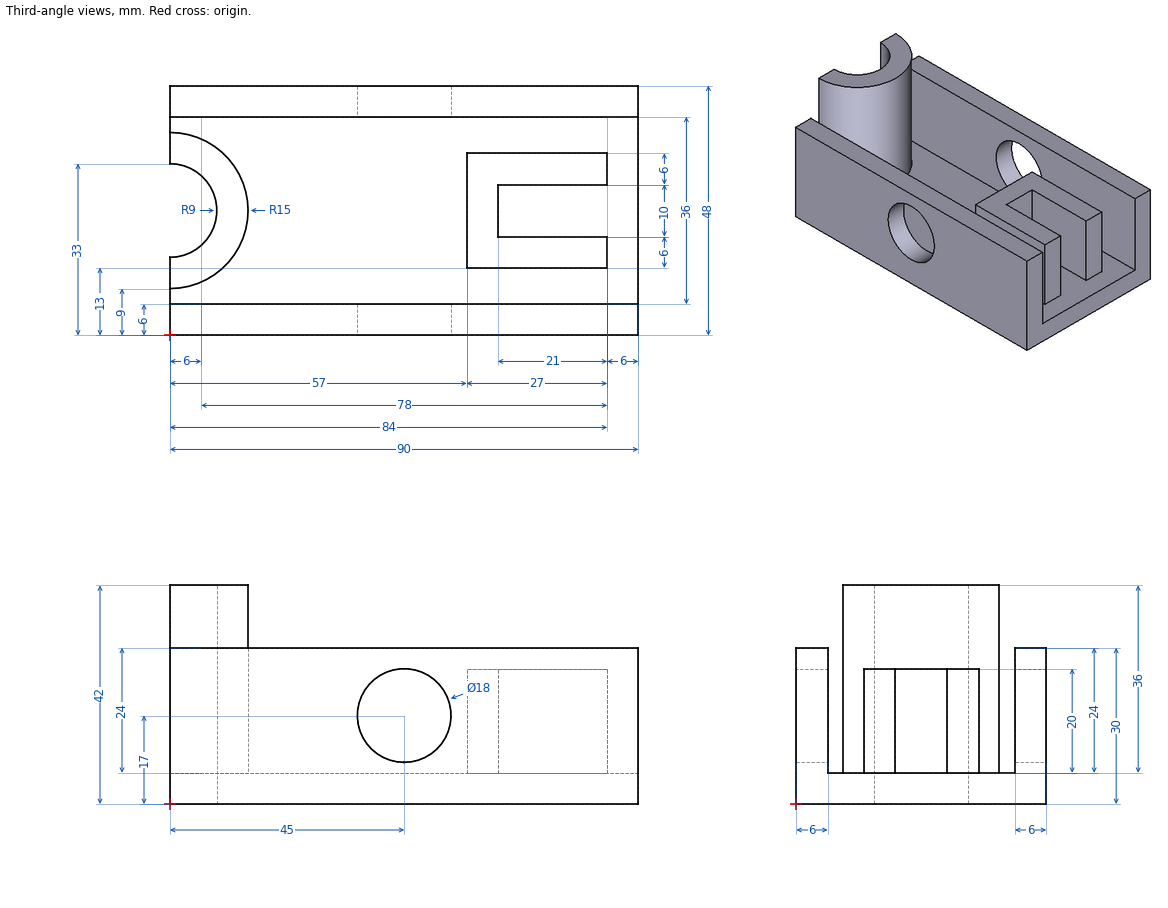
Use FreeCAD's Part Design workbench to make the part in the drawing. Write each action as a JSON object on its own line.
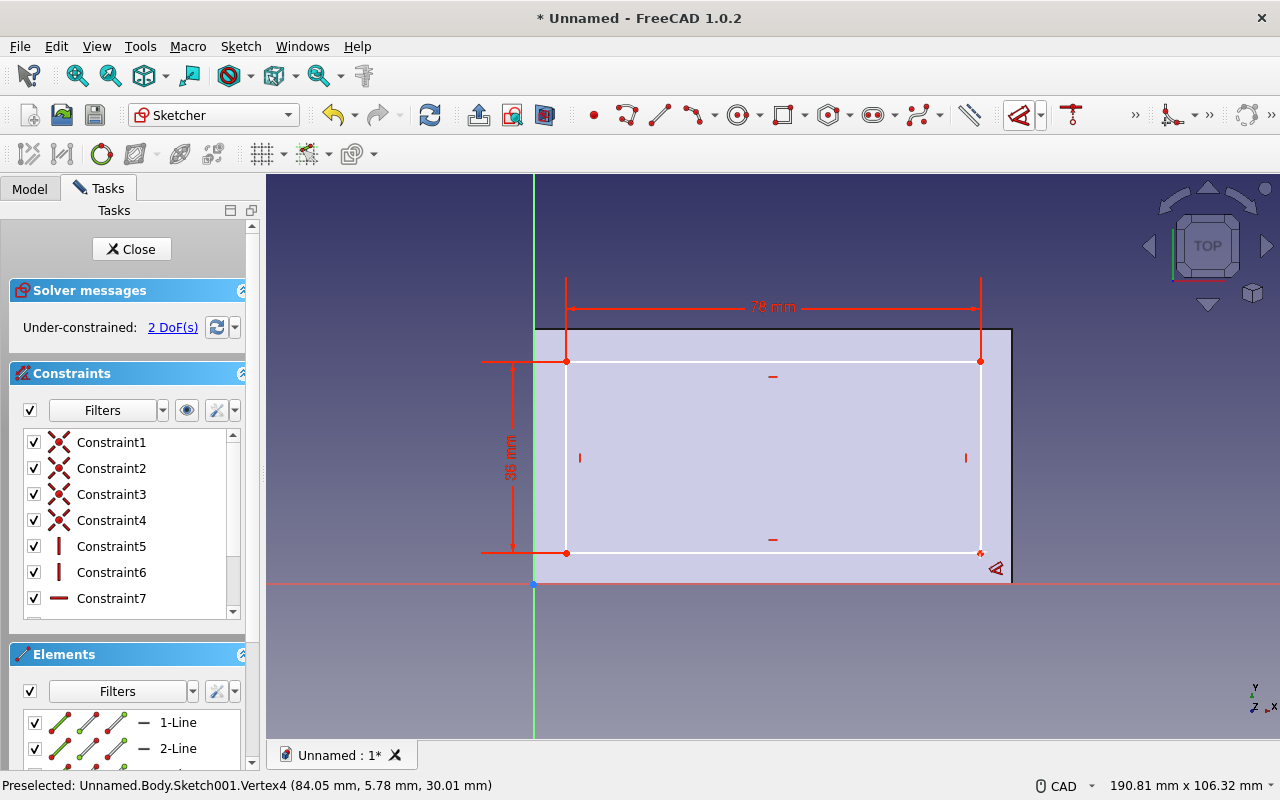
{"action": "scroll", "coordinate": [566, 362], "scroll_direction": "up", "scroll_amount": 2}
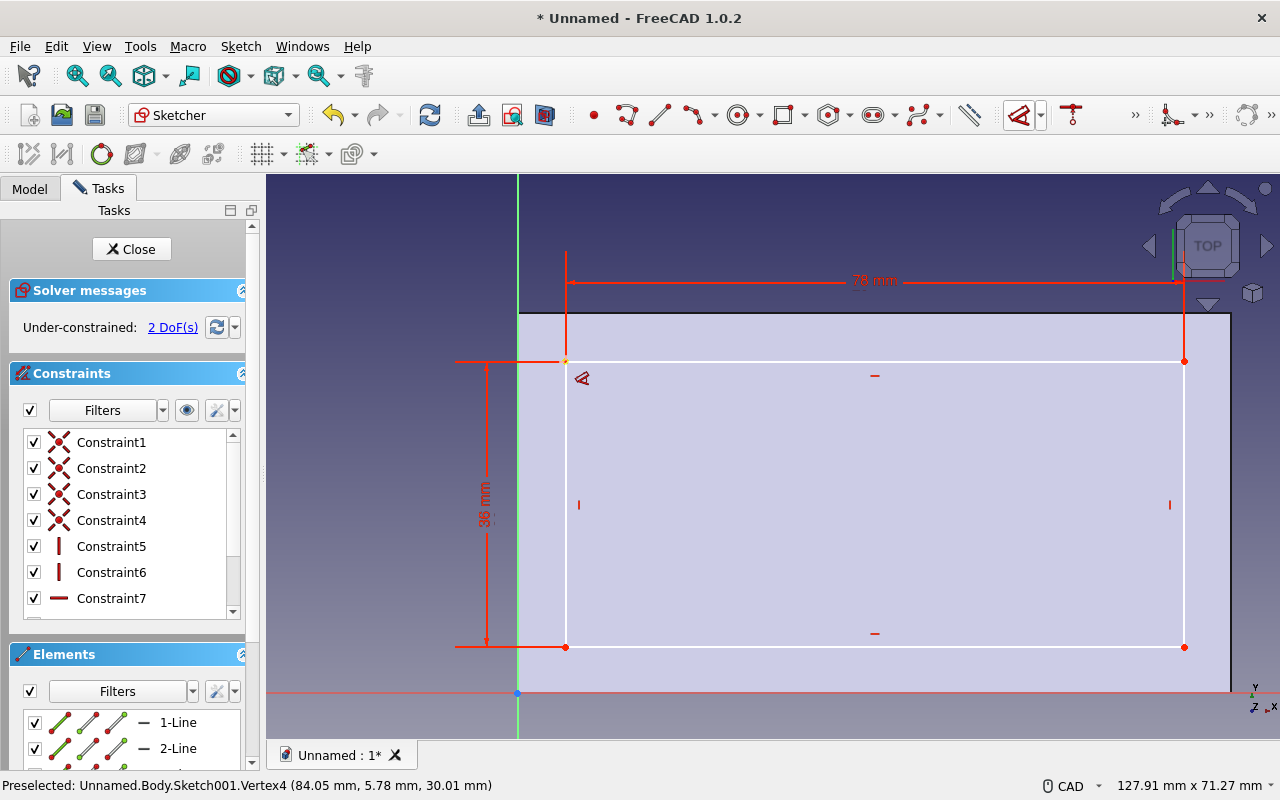
{"action": "left_click", "coordinate": [566, 362]}
{"action": "left_click", "coordinate": [542, 328]}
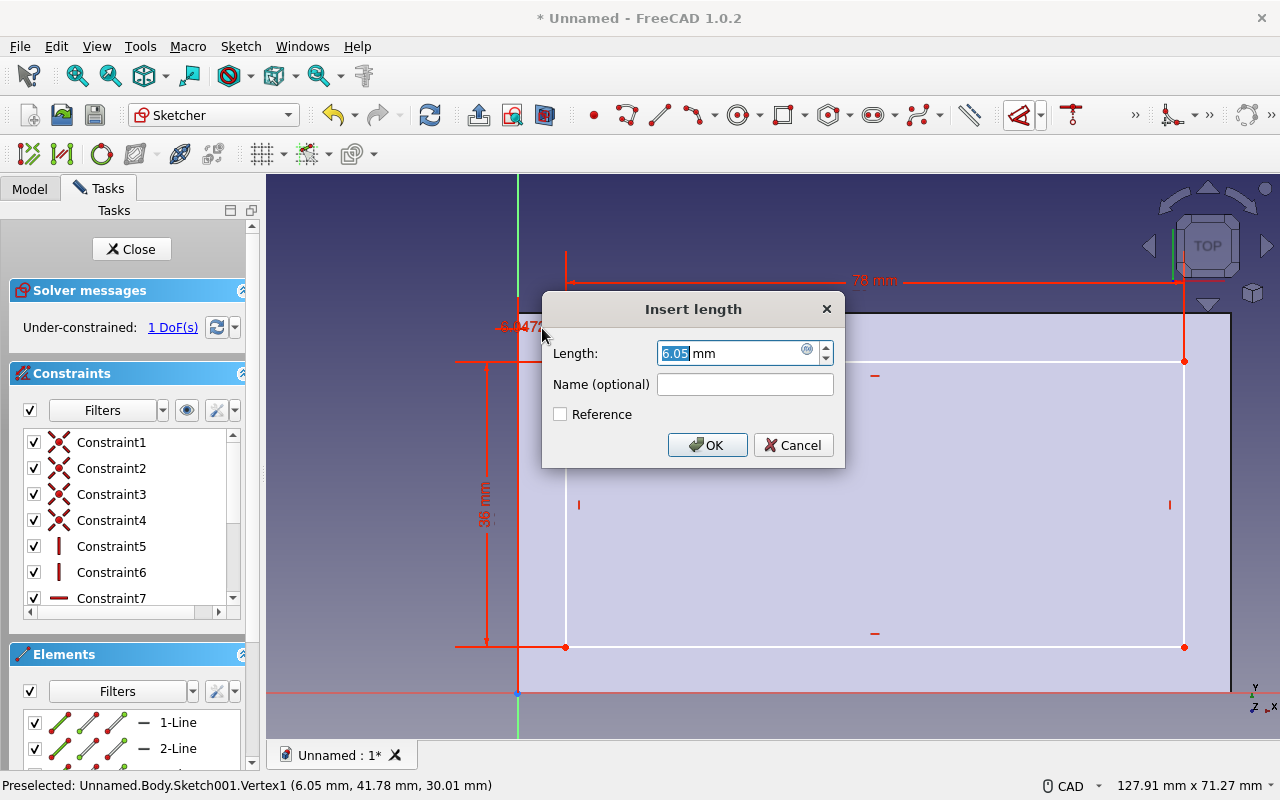
{"action": "type", "text": "6"}
{"action": "key", "text": "Return"}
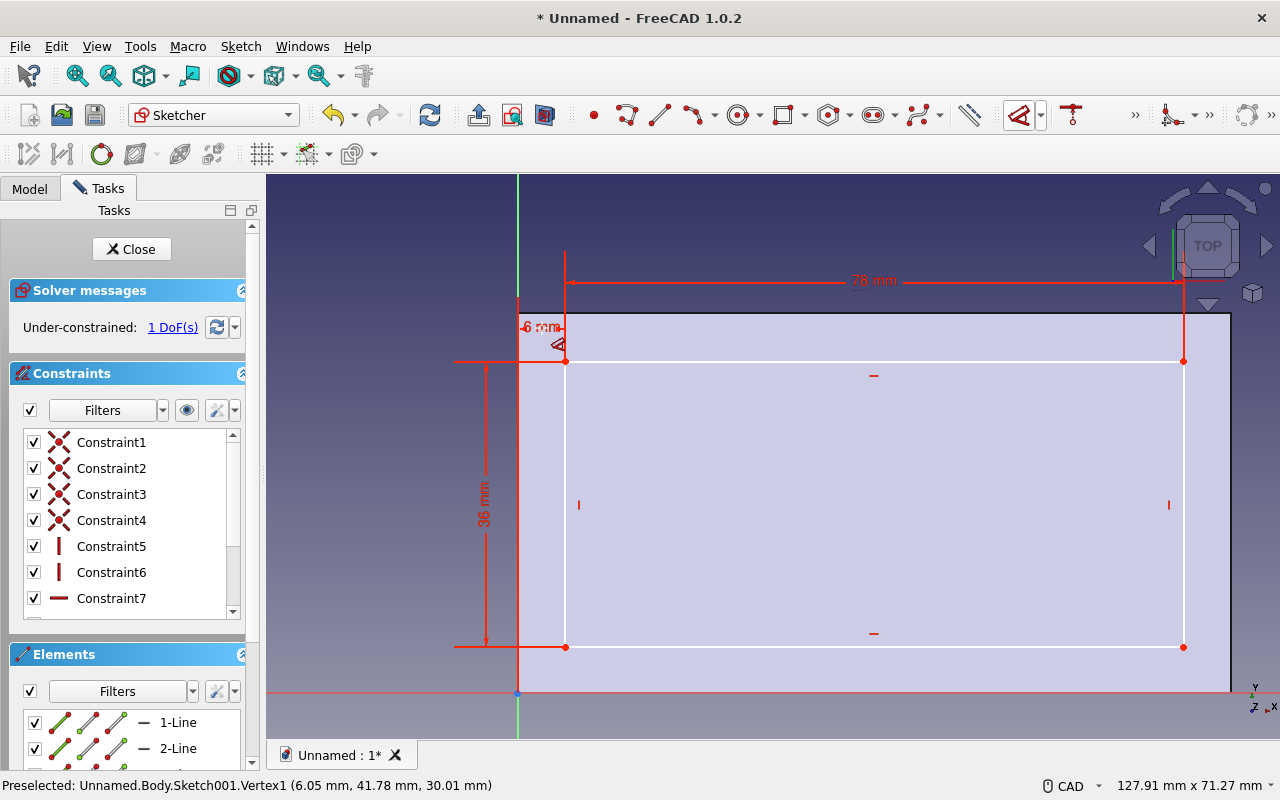
{"action": "left_click", "coordinate": [565, 647]}
{"action": "left_click", "coordinate": [484, 670]}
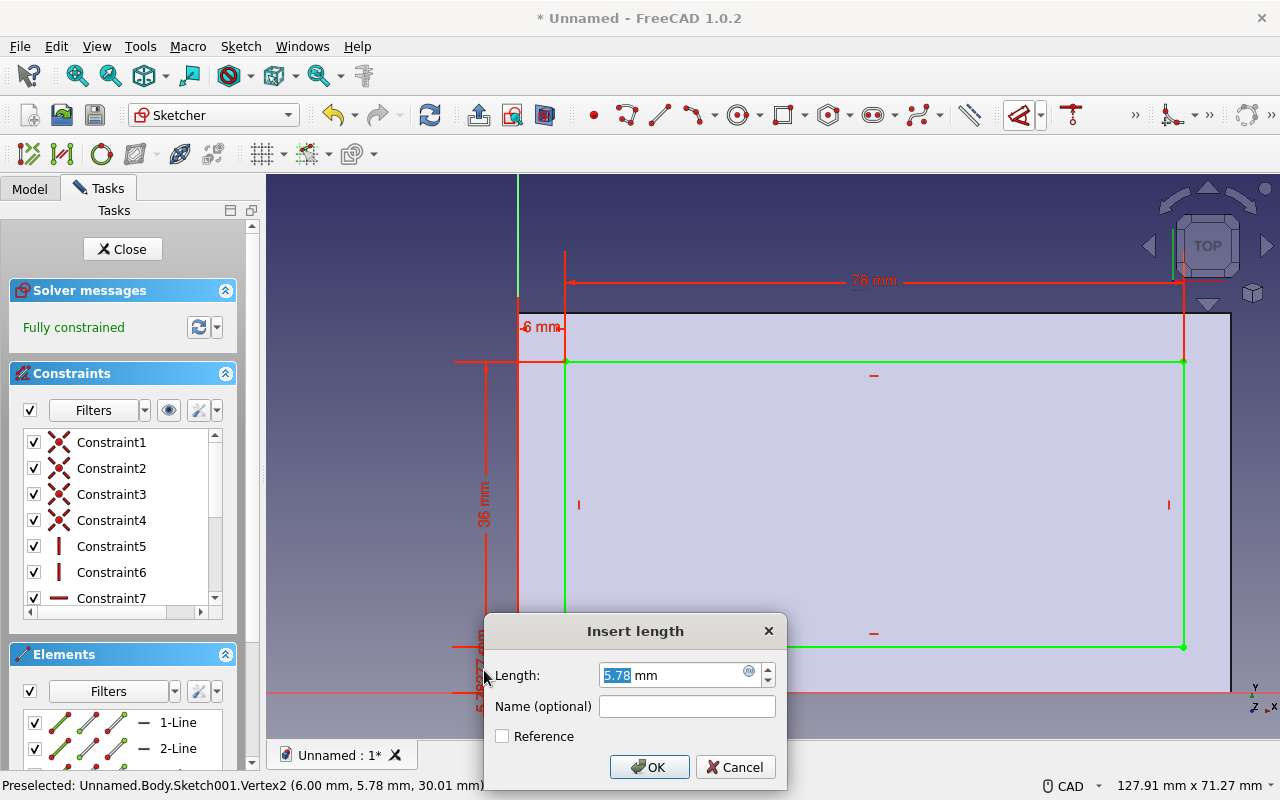
{"action": "type", "text": "6"}
{"action": "key", "text": "Return"}
{"action": "key", "text": "Escape"}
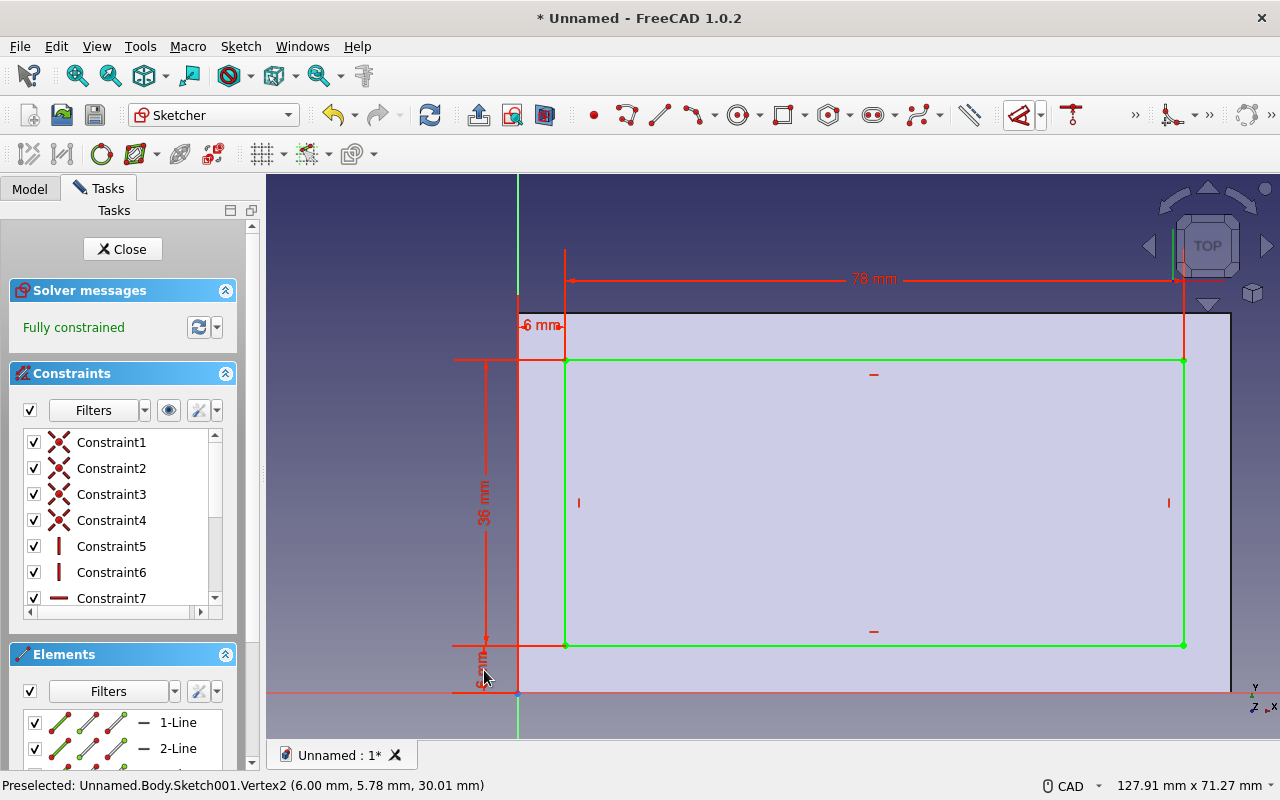
{"action": "left_click", "coordinate": [123, 249]}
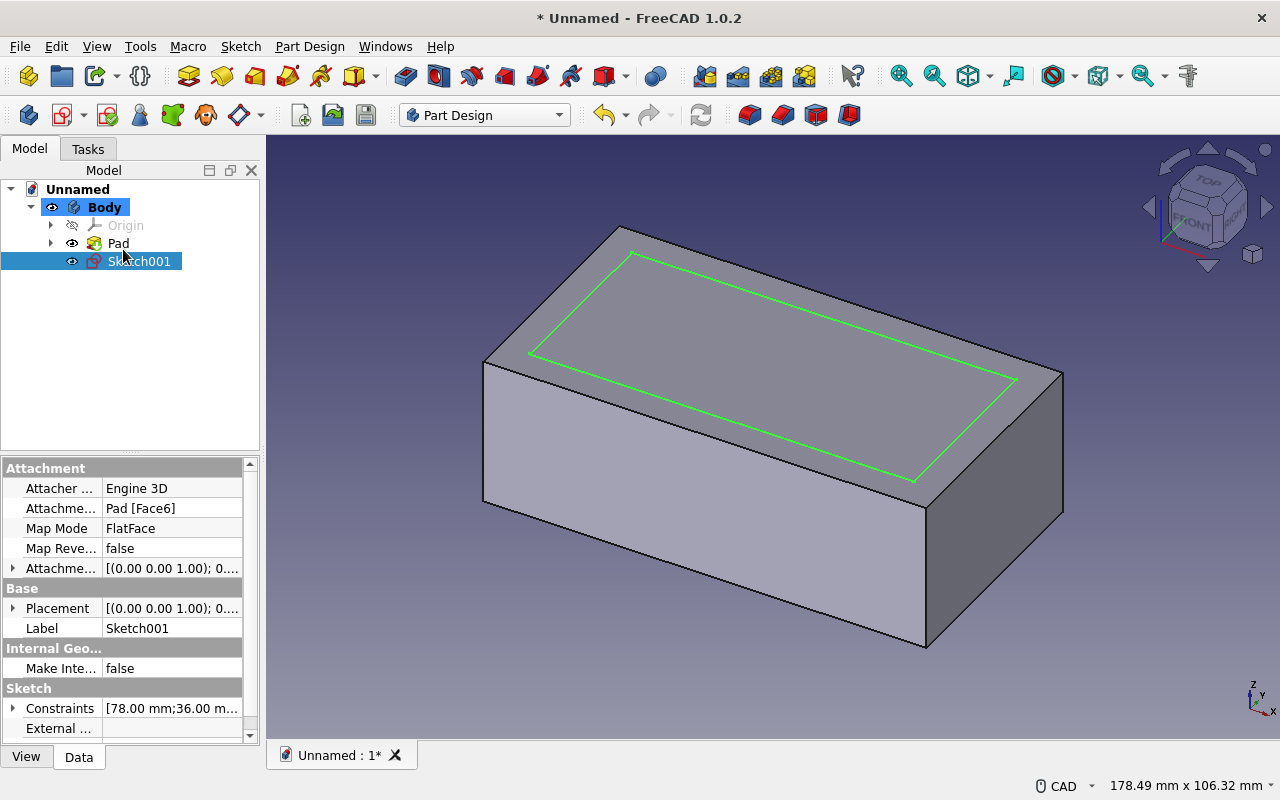
{"action": "left_click", "coordinate": [406, 76]}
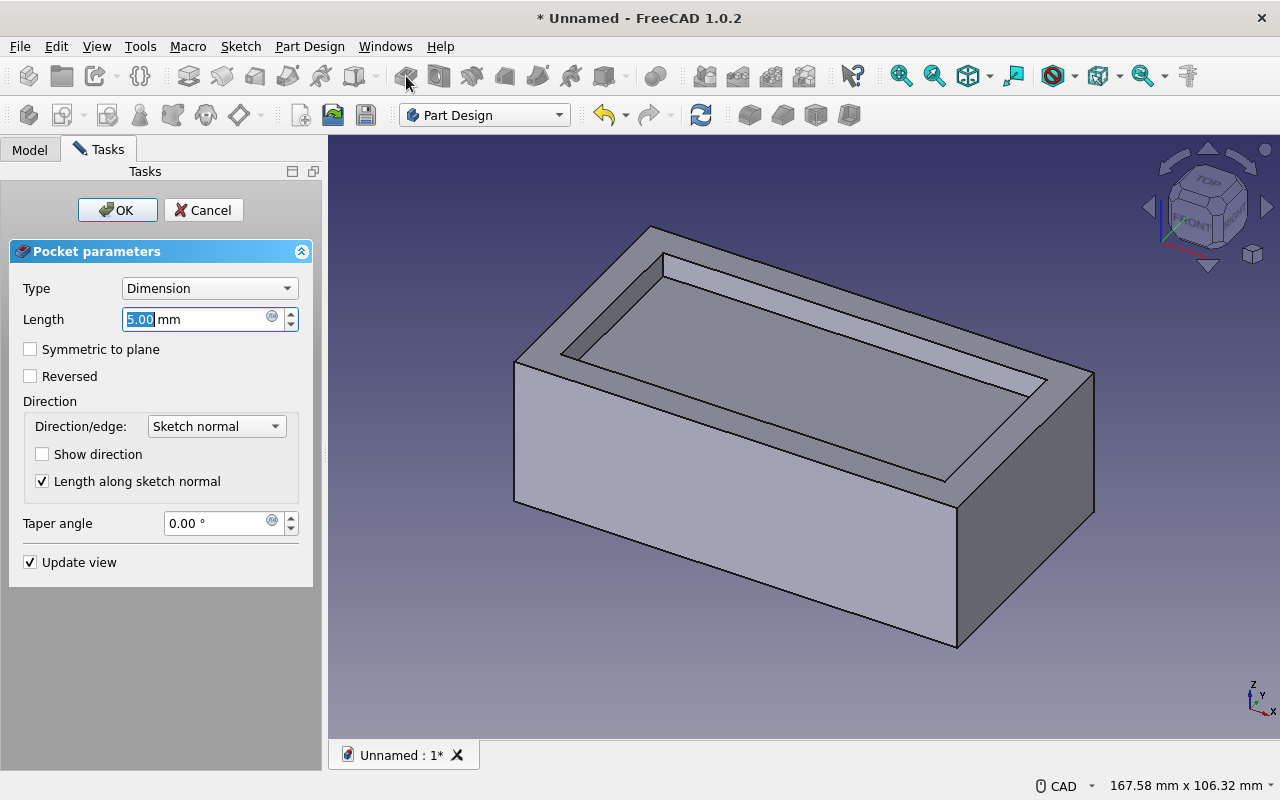
{"action": "type", "text": "24"}
{"action": "key", "text": "Tab"}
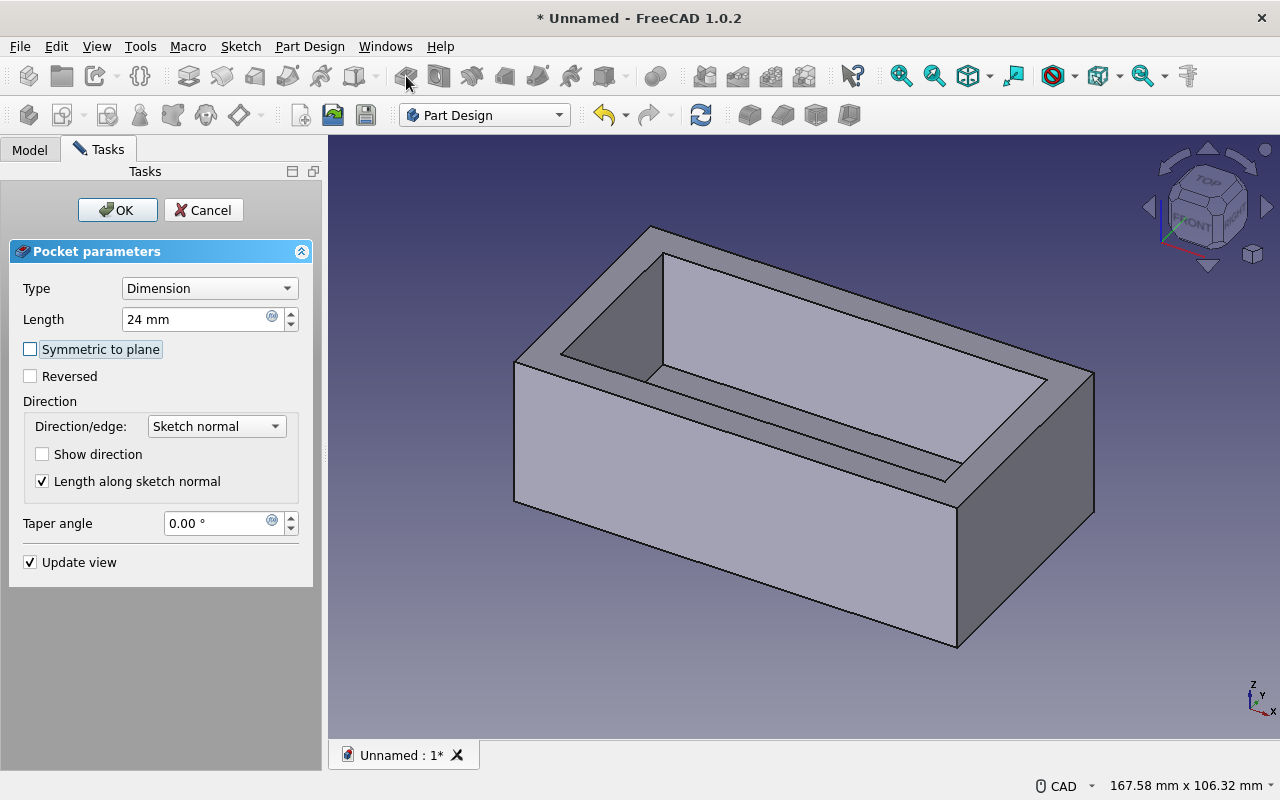
{"action": "left_click", "coordinate": [118, 210]}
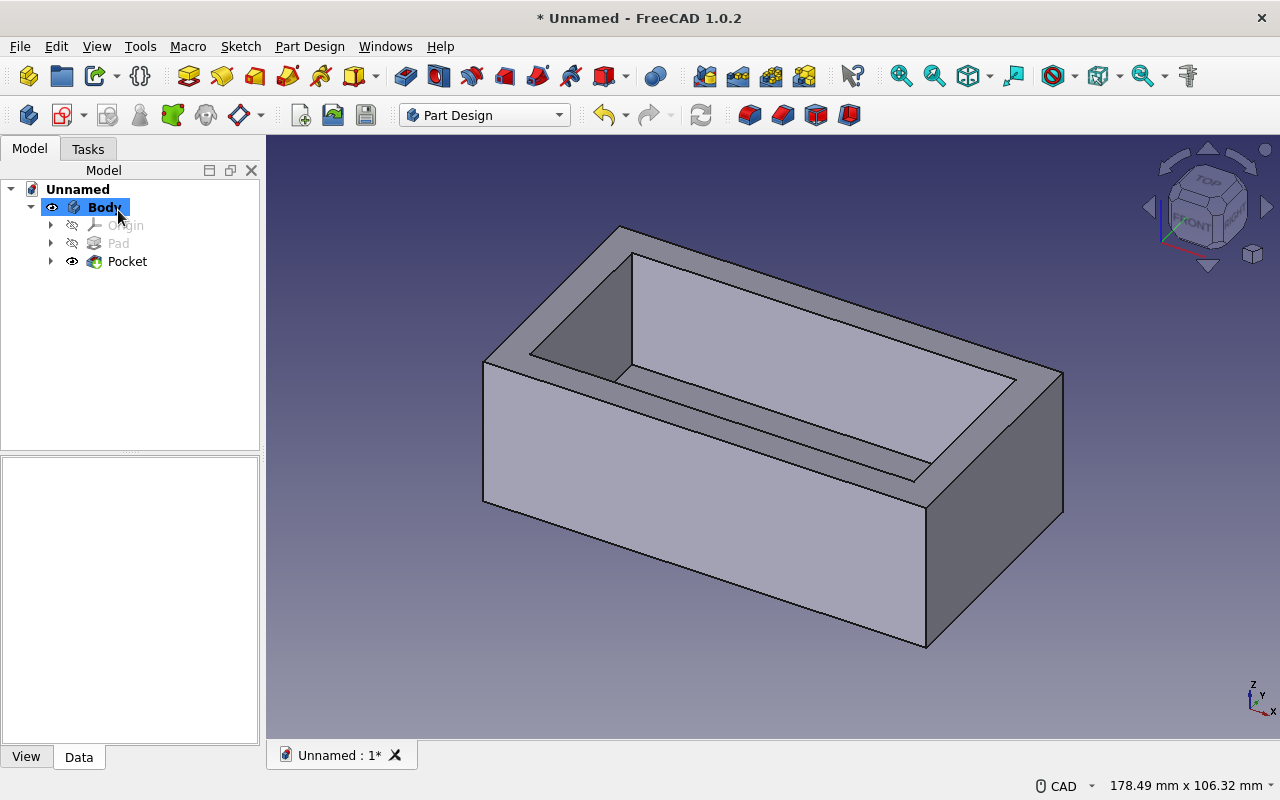
{"action": "left_click", "coordinate": [904, 487]}